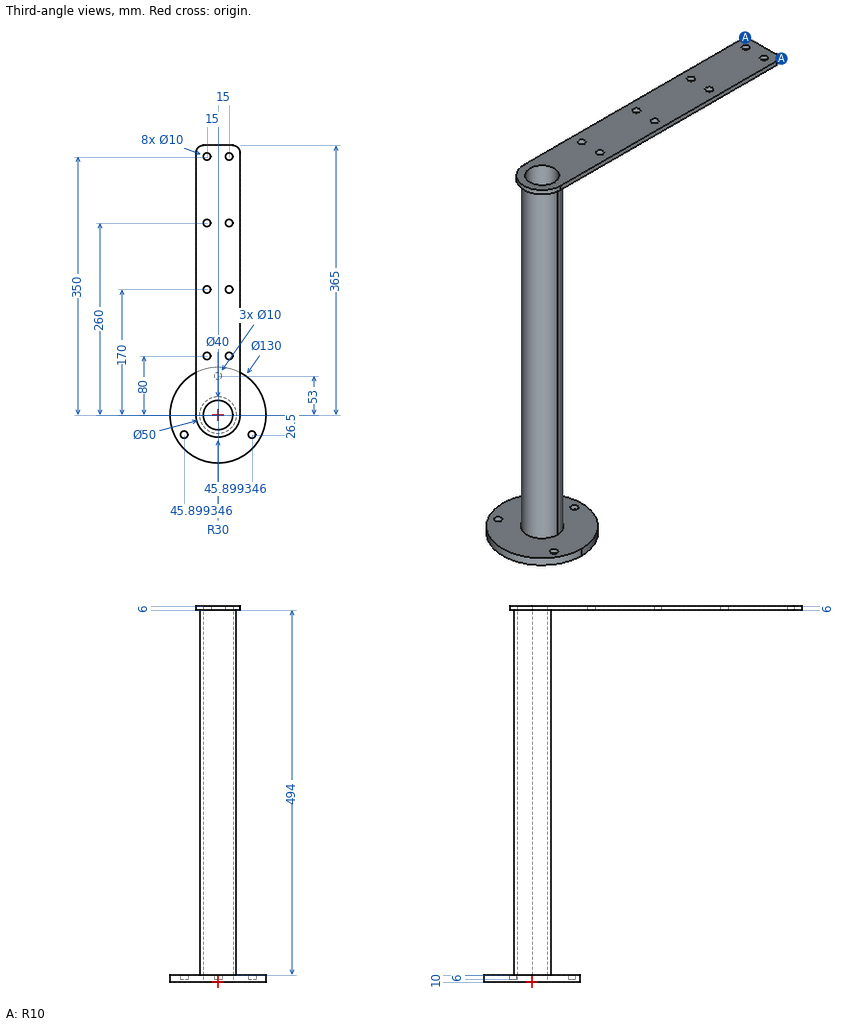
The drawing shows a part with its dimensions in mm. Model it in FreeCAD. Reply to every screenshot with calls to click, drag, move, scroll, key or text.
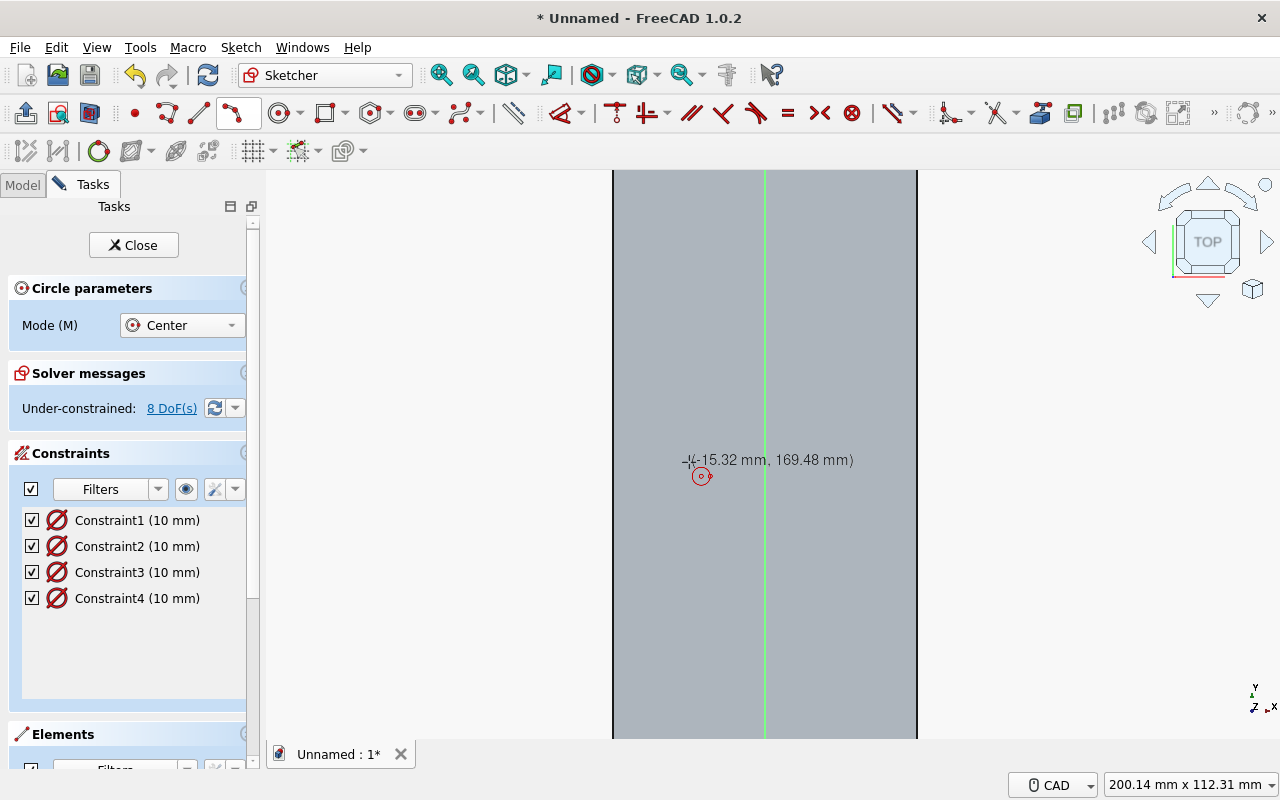
scroll(689, 462, down, 8)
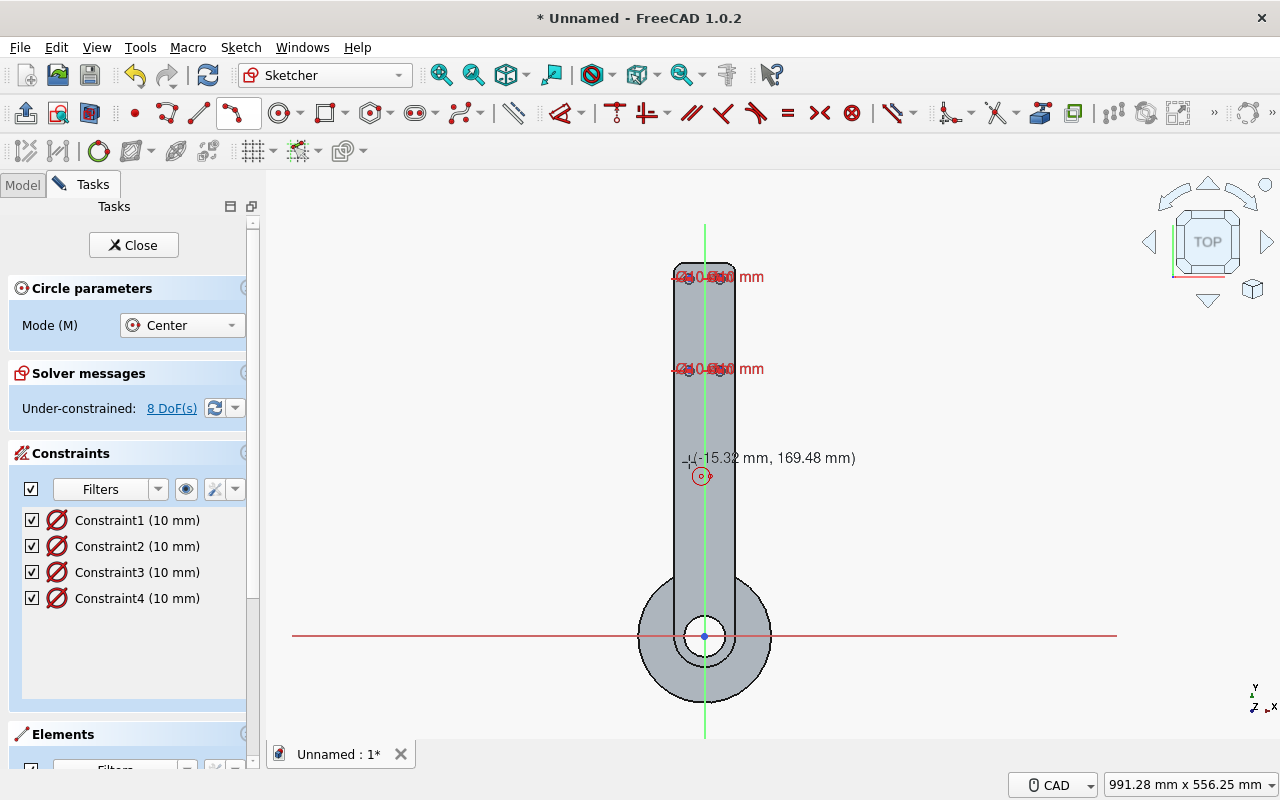
click(689, 462)
move(686, 459)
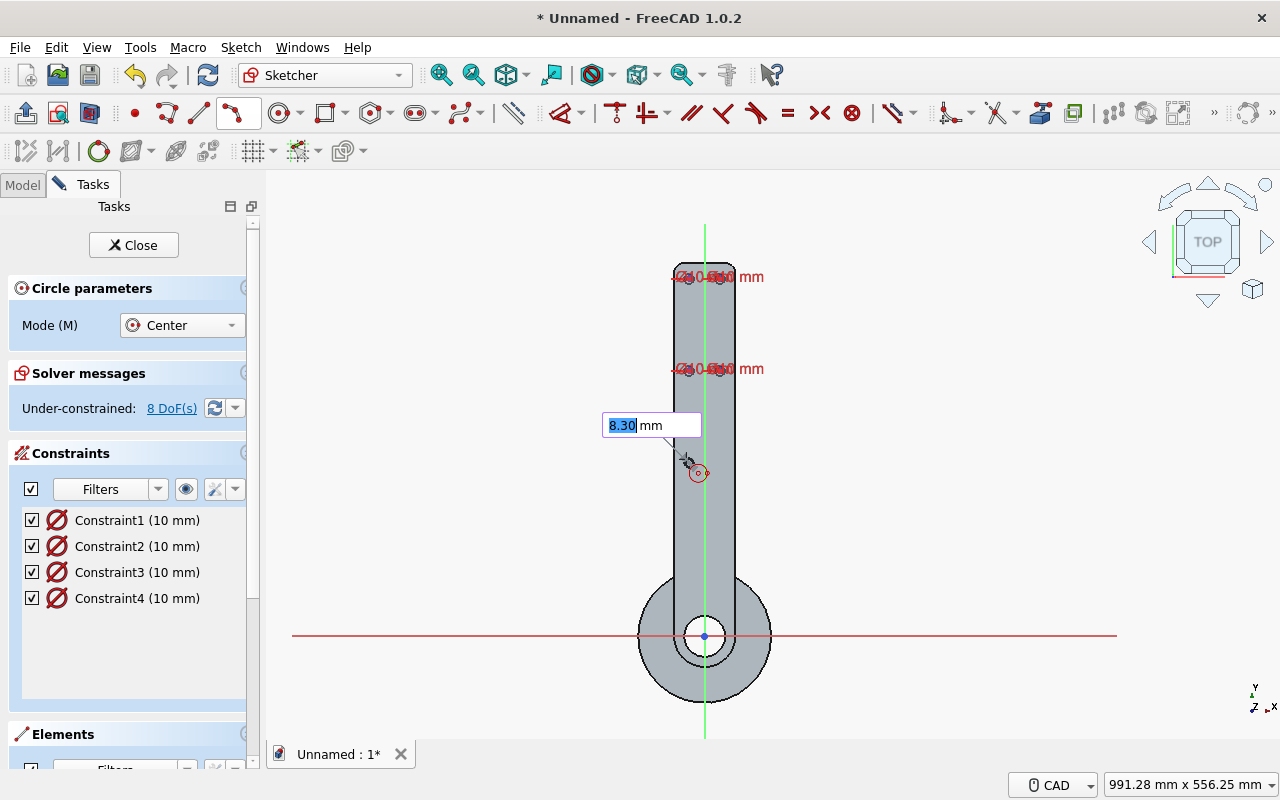
text(10)
key(Return)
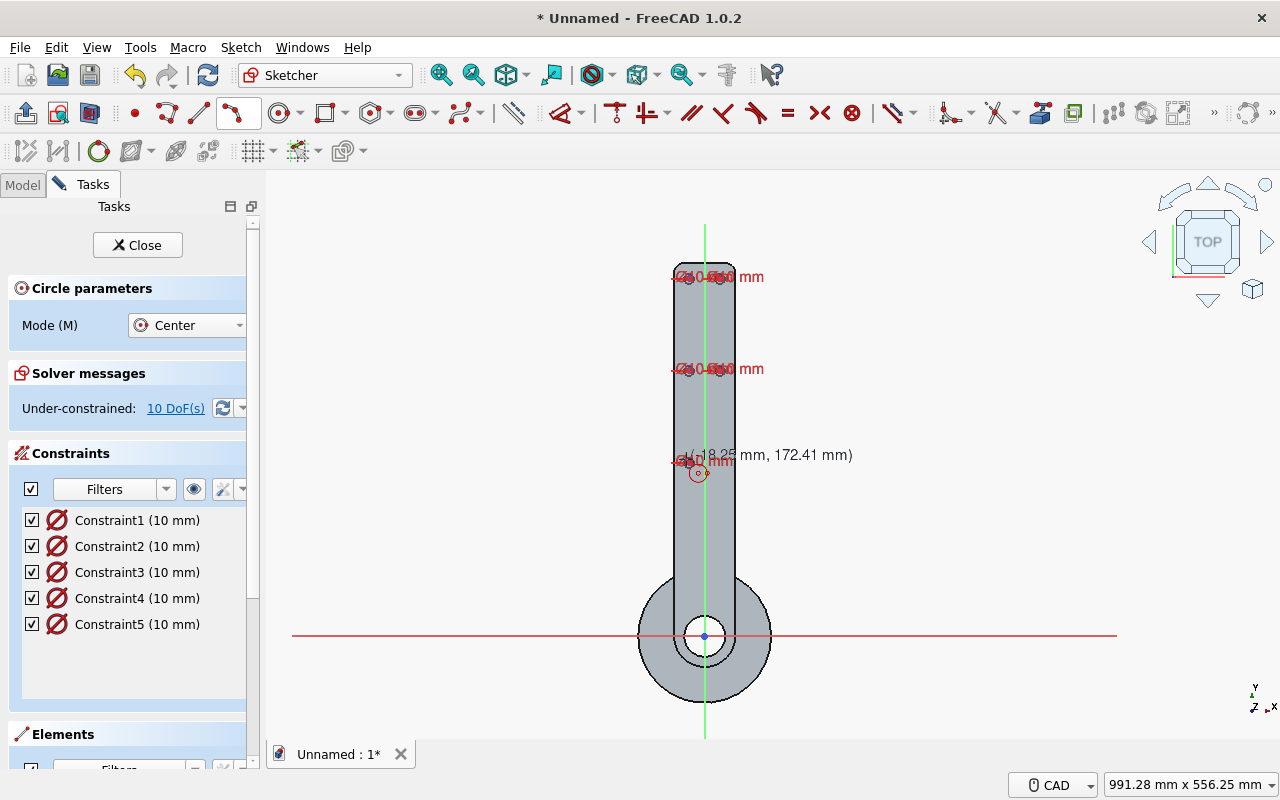
scroll(720, 462, up, 8)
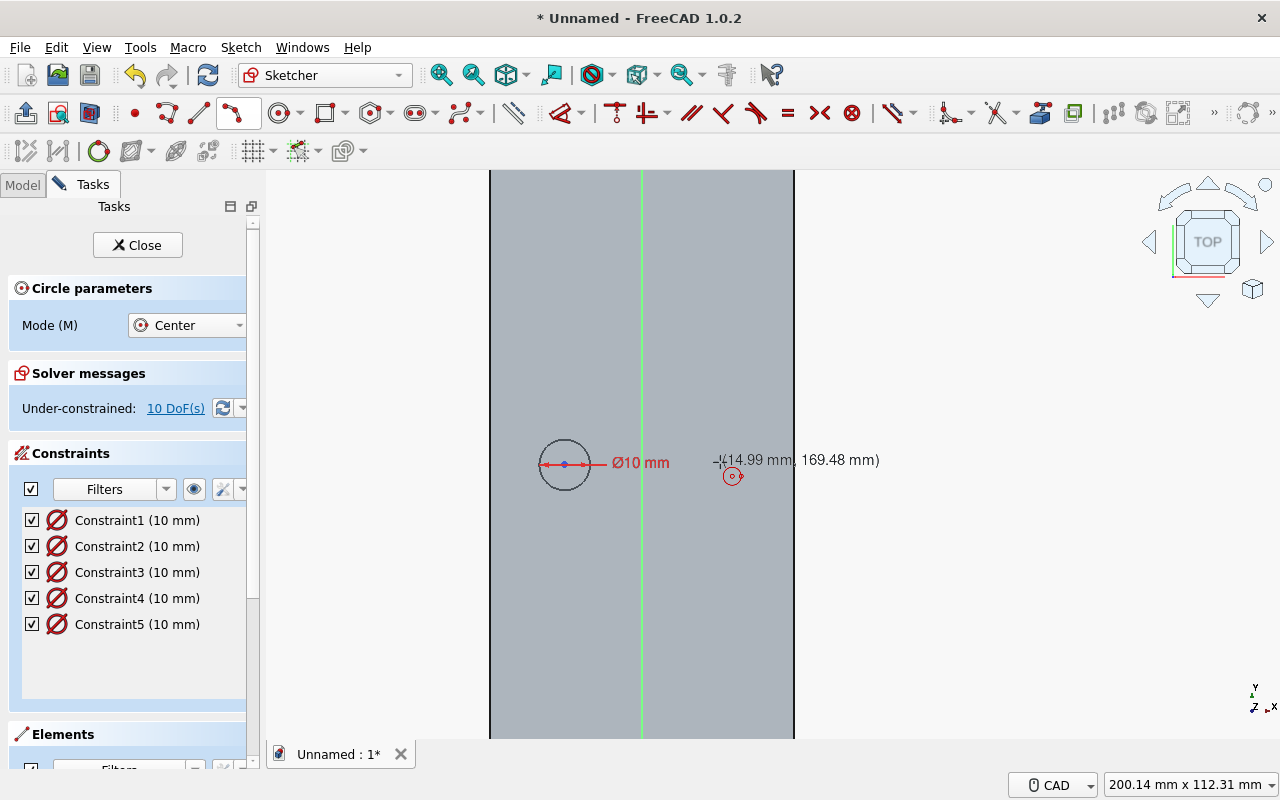
scroll(720, 462, down, 8)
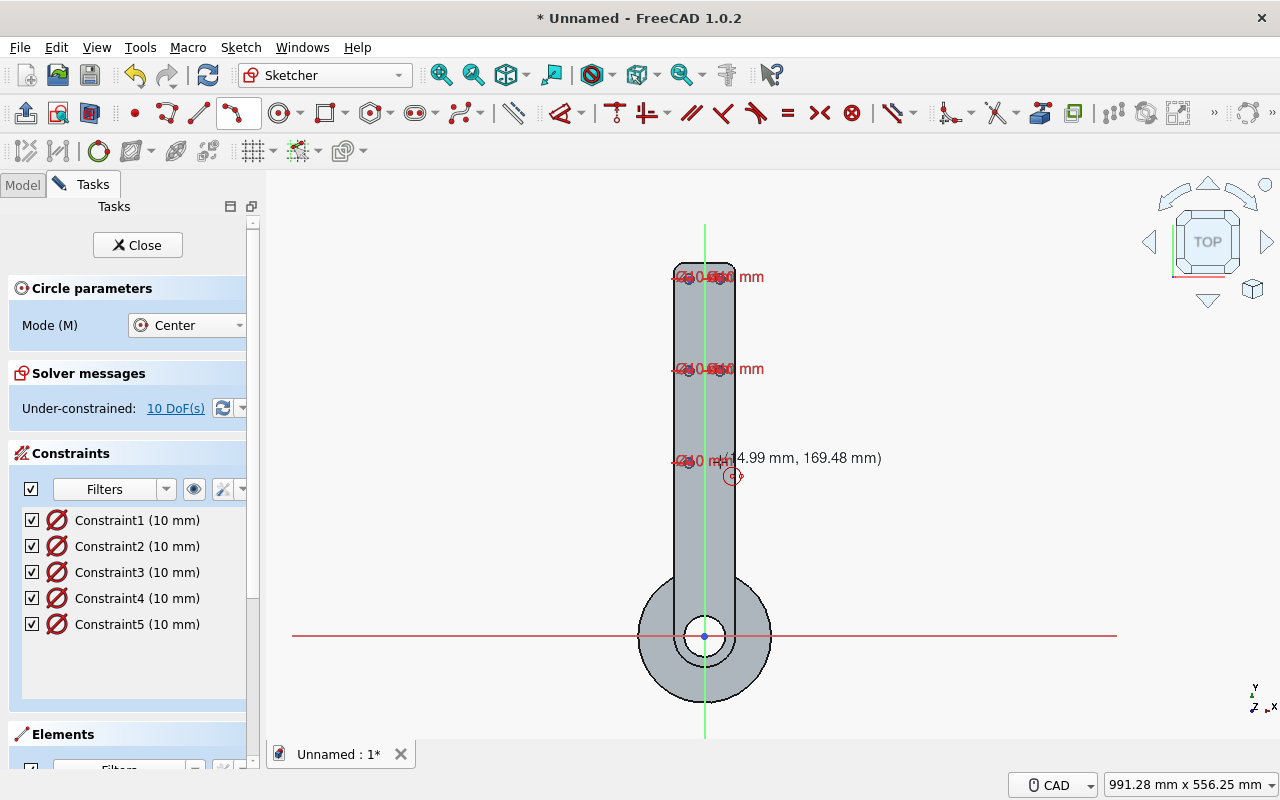
click(720, 462)
move(724, 459)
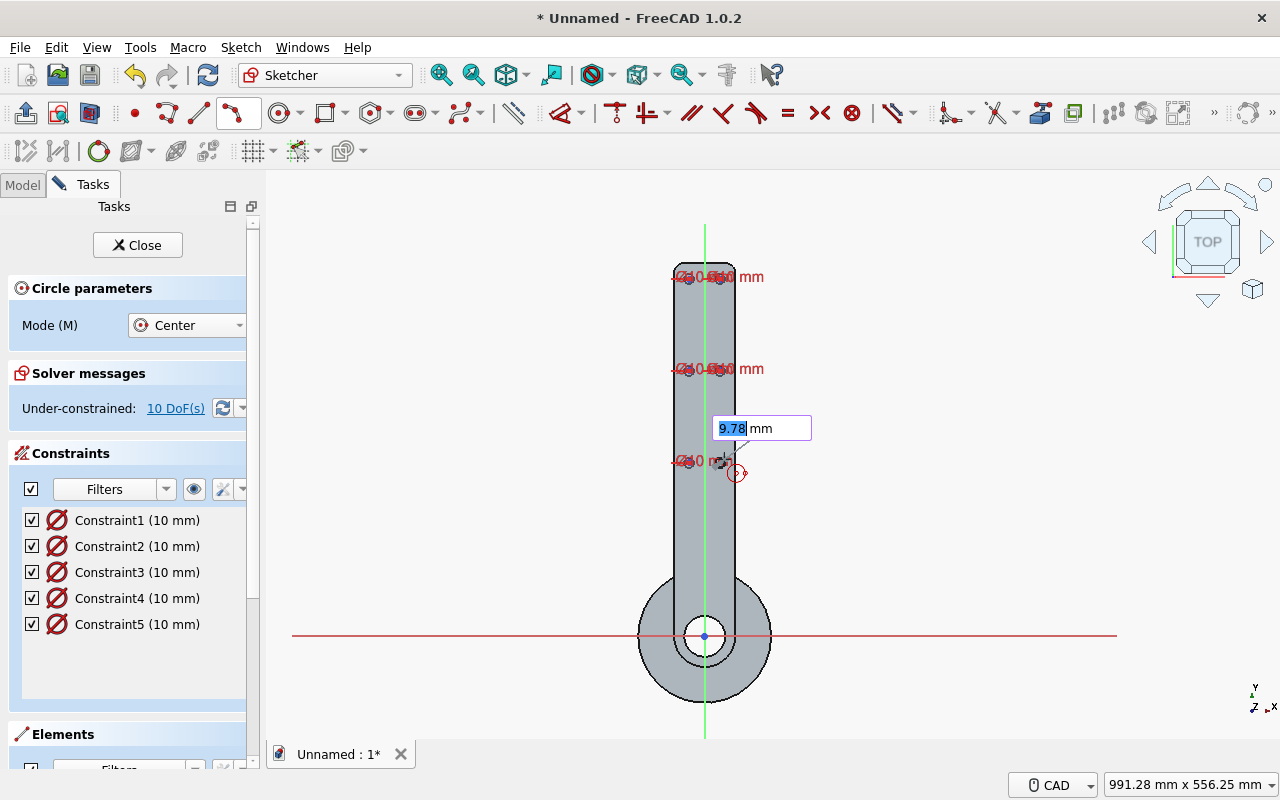
text(10)
key(Return)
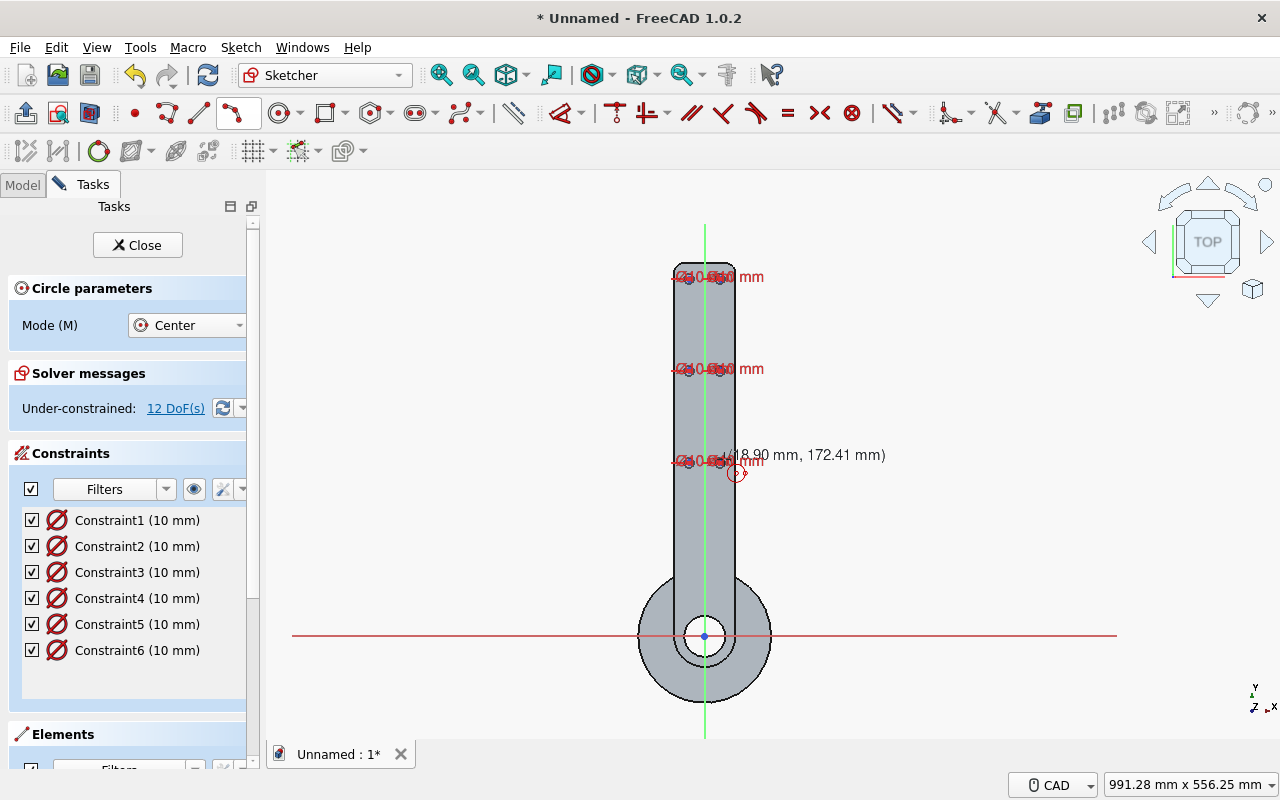
scroll(689, 555, up, 8)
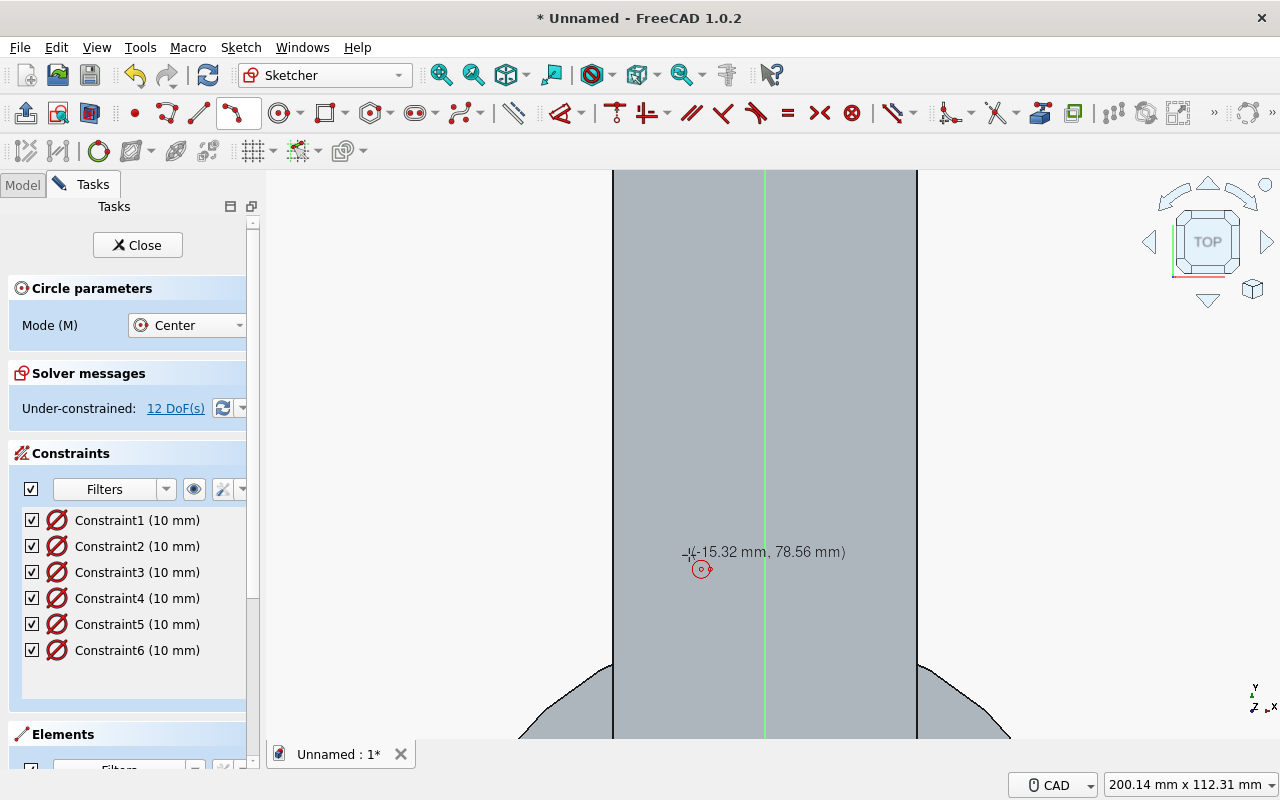
scroll(689, 555, down, 8)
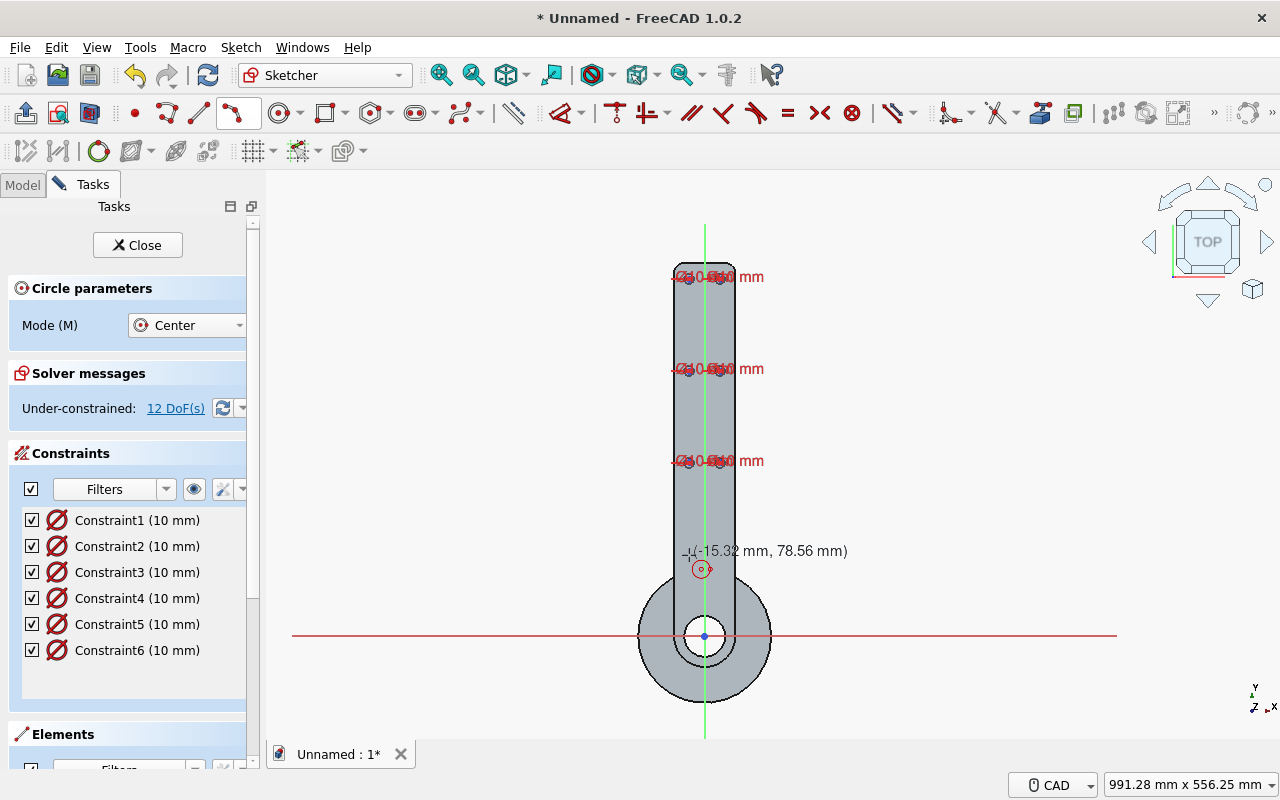
click(689, 555)
move(686, 551)